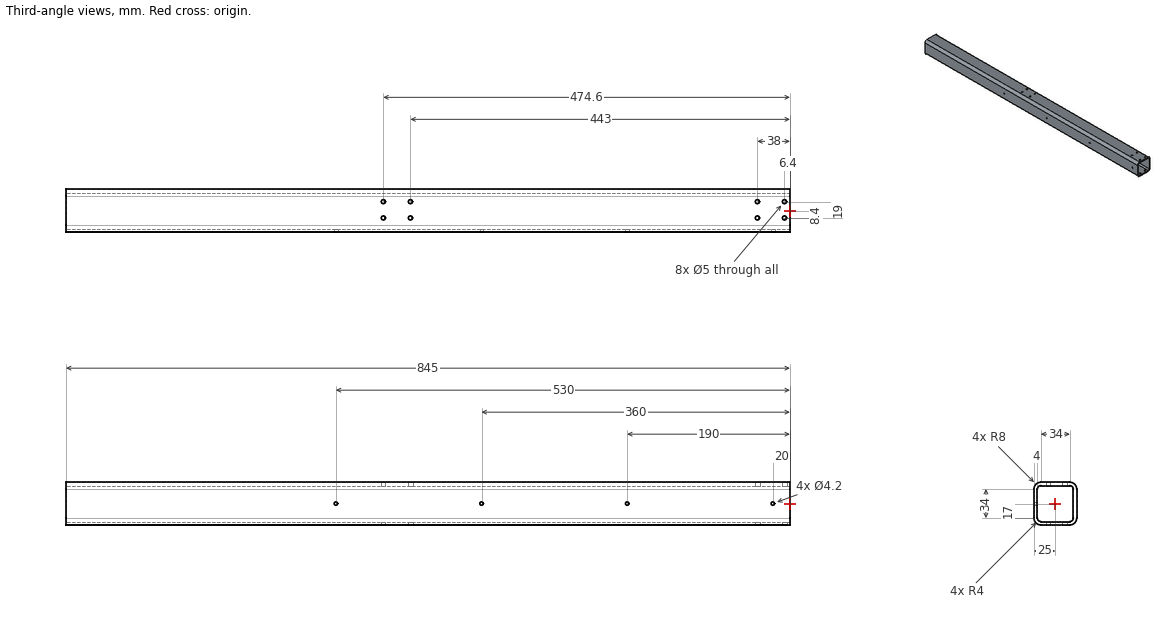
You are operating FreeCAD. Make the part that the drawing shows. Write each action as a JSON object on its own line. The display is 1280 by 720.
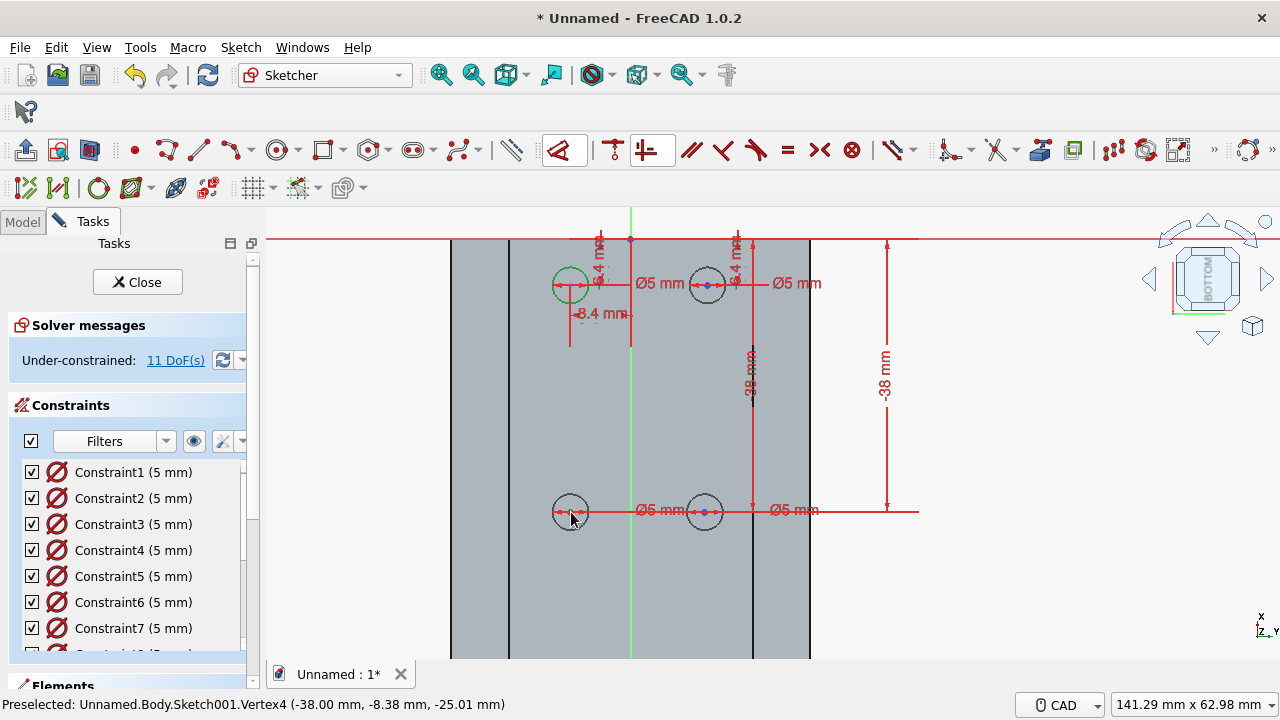
{"action": "left_click", "coordinate": [582, 150]}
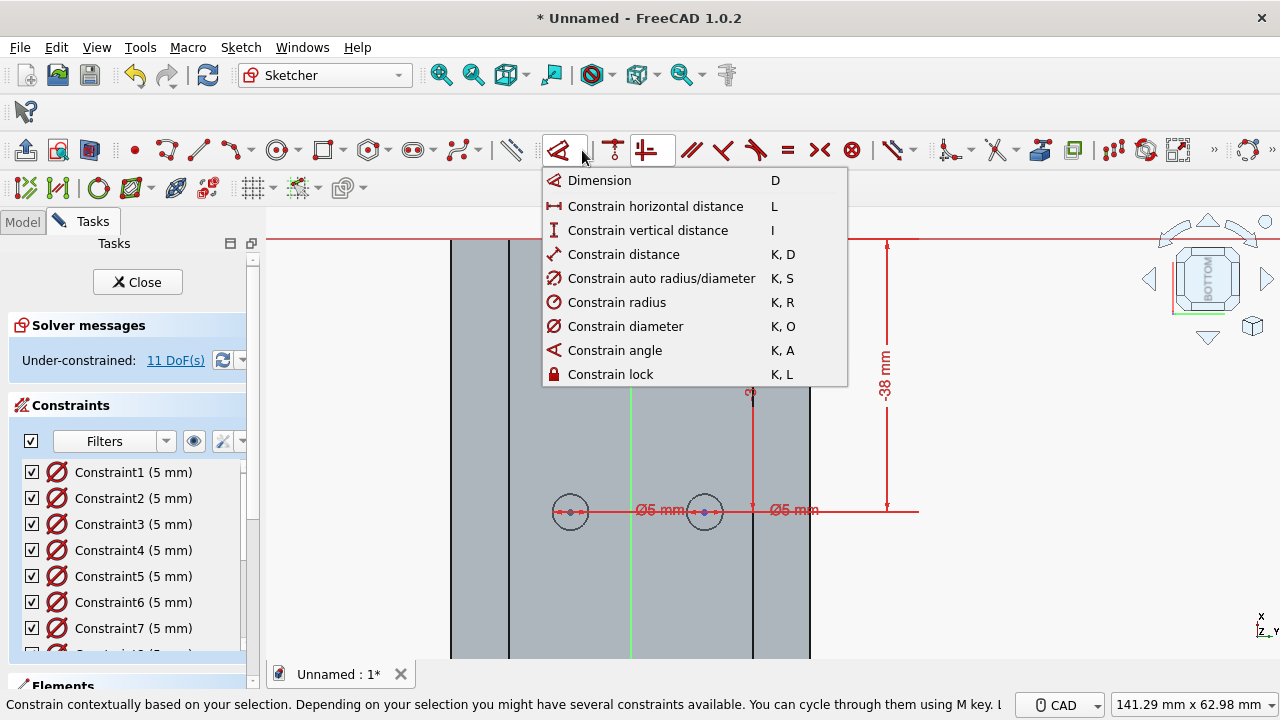
{"action": "left_click", "coordinate": [695, 206]}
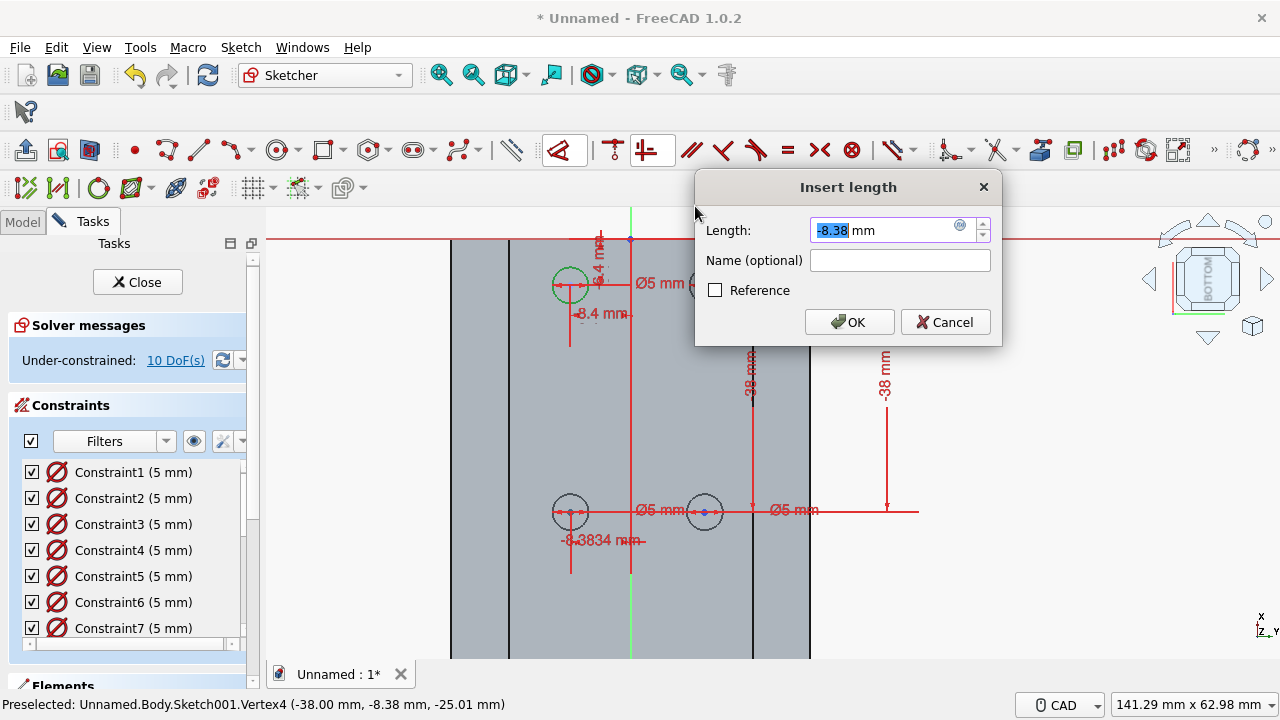
{"action": "type", "text": "-8.4"}
{"action": "key", "text": "Return"}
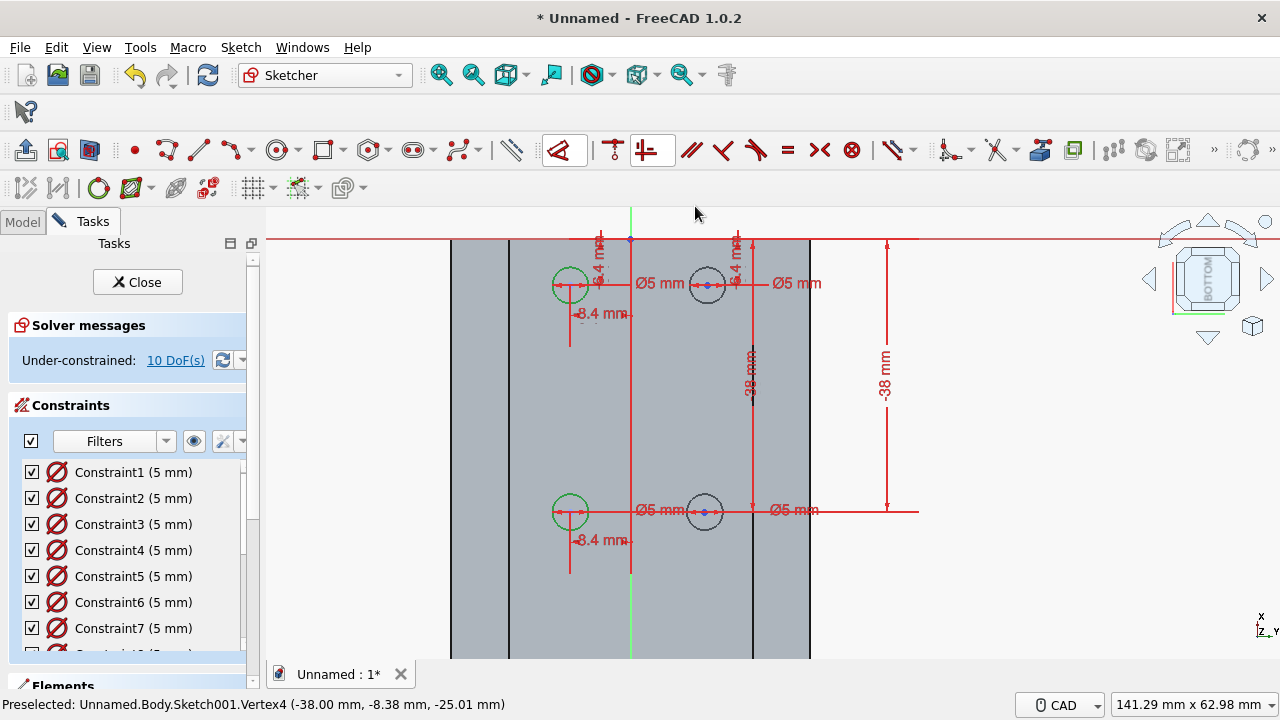
{"action": "scroll", "coordinate": [710, 311], "scroll_direction": "down", "scroll_amount": 13}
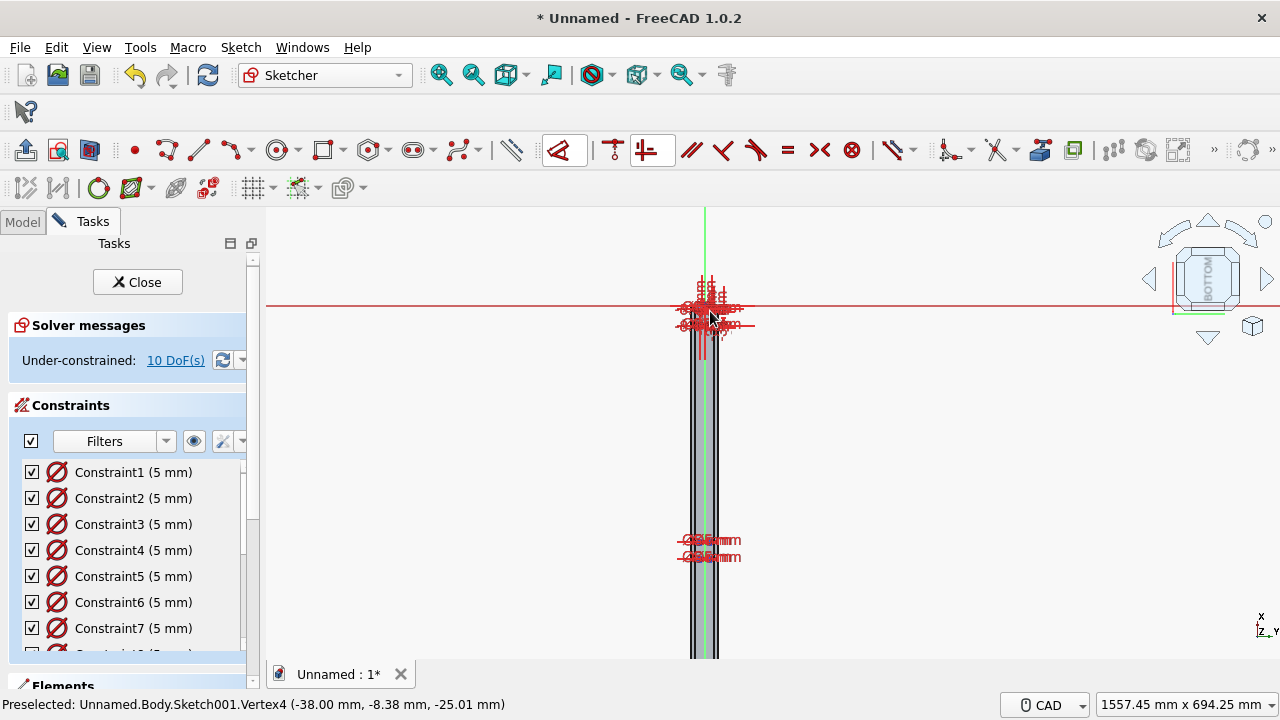
{"action": "left_click", "coordinate": [710, 542]}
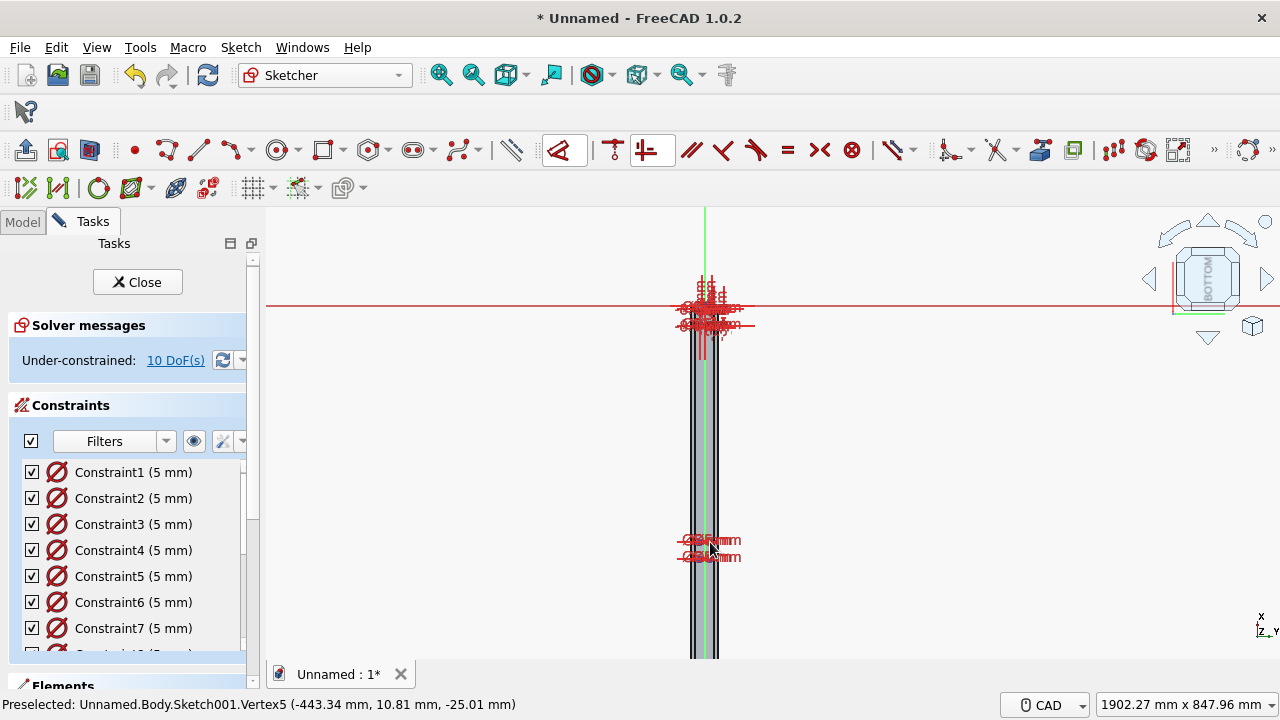
{"action": "left_click", "coordinate": [582, 150]}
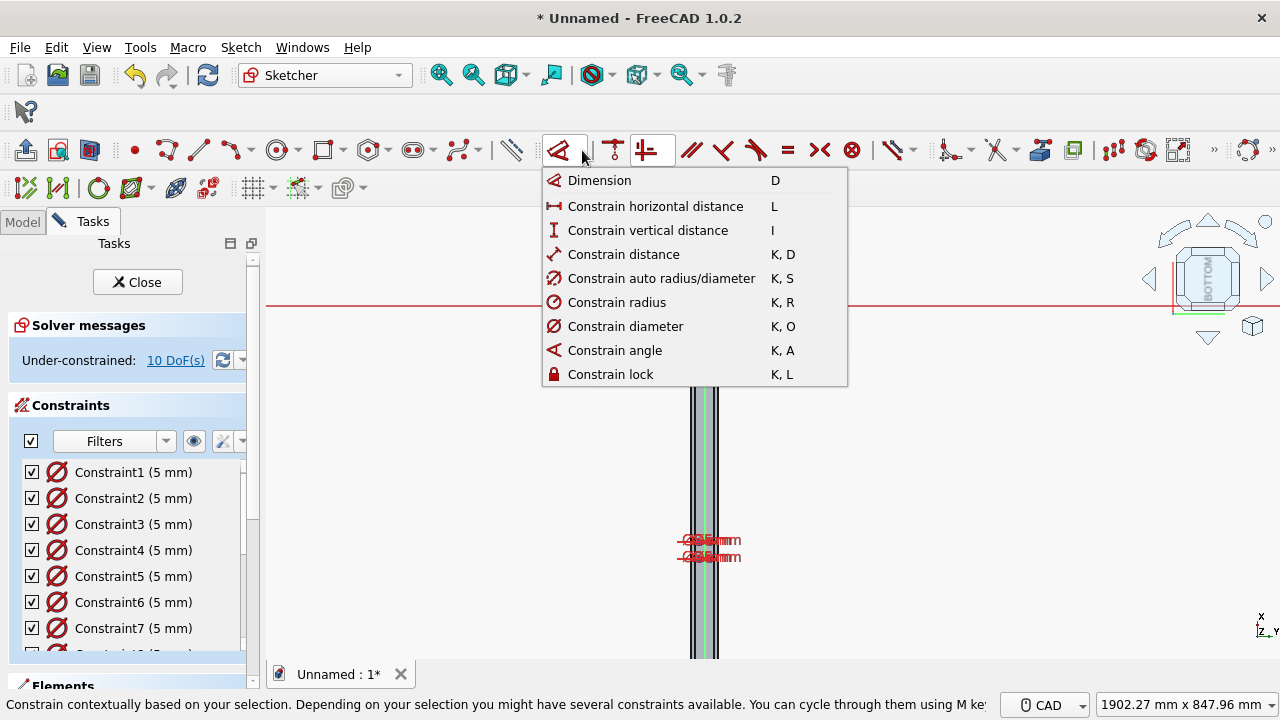
{"action": "left_click", "coordinate": [695, 230]}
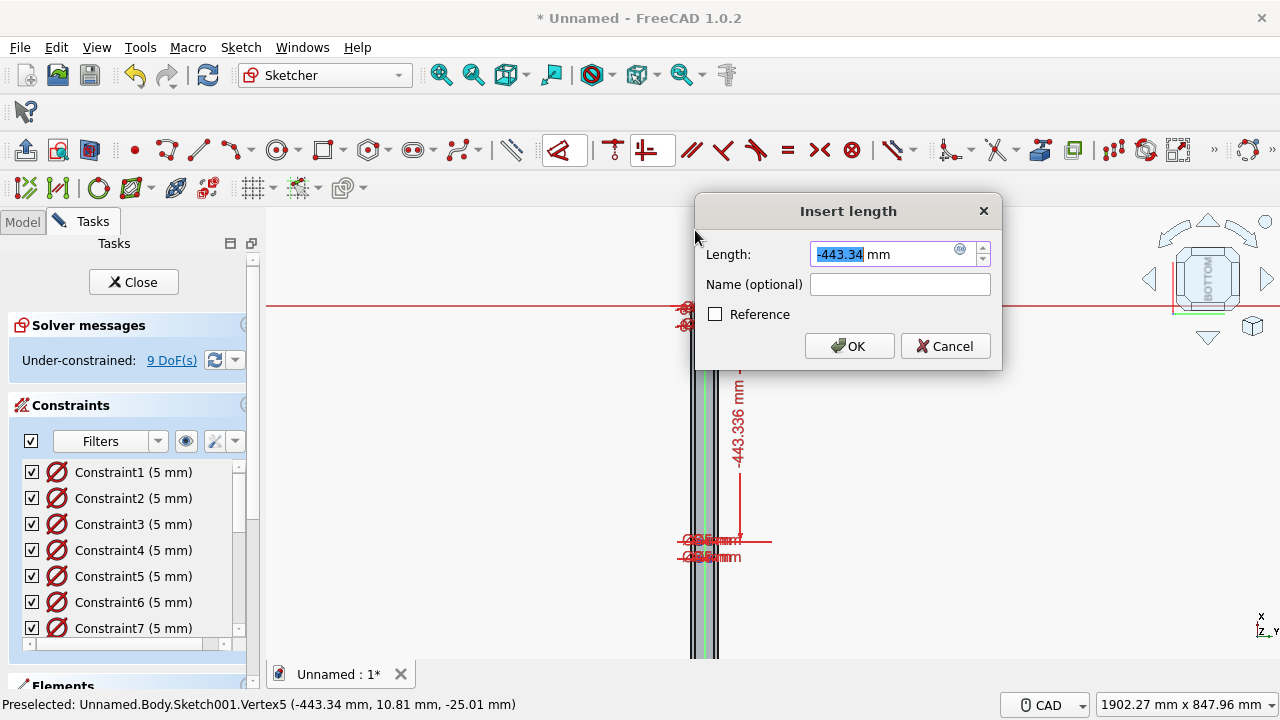
{"action": "type", "text": "-443"}
{"action": "key", "text": "Return"}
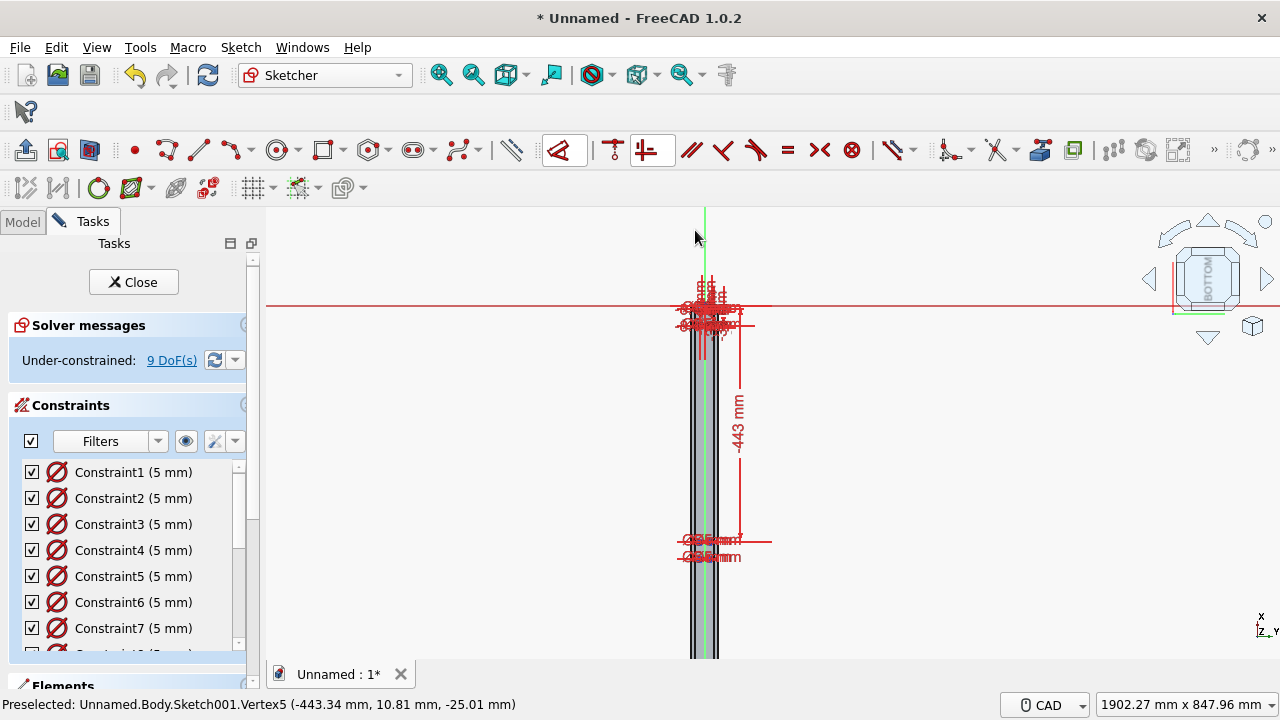
{"action": "scroll", "coordinate": [700, 542], "scroll_direction": "up", "scroll_amount": 11}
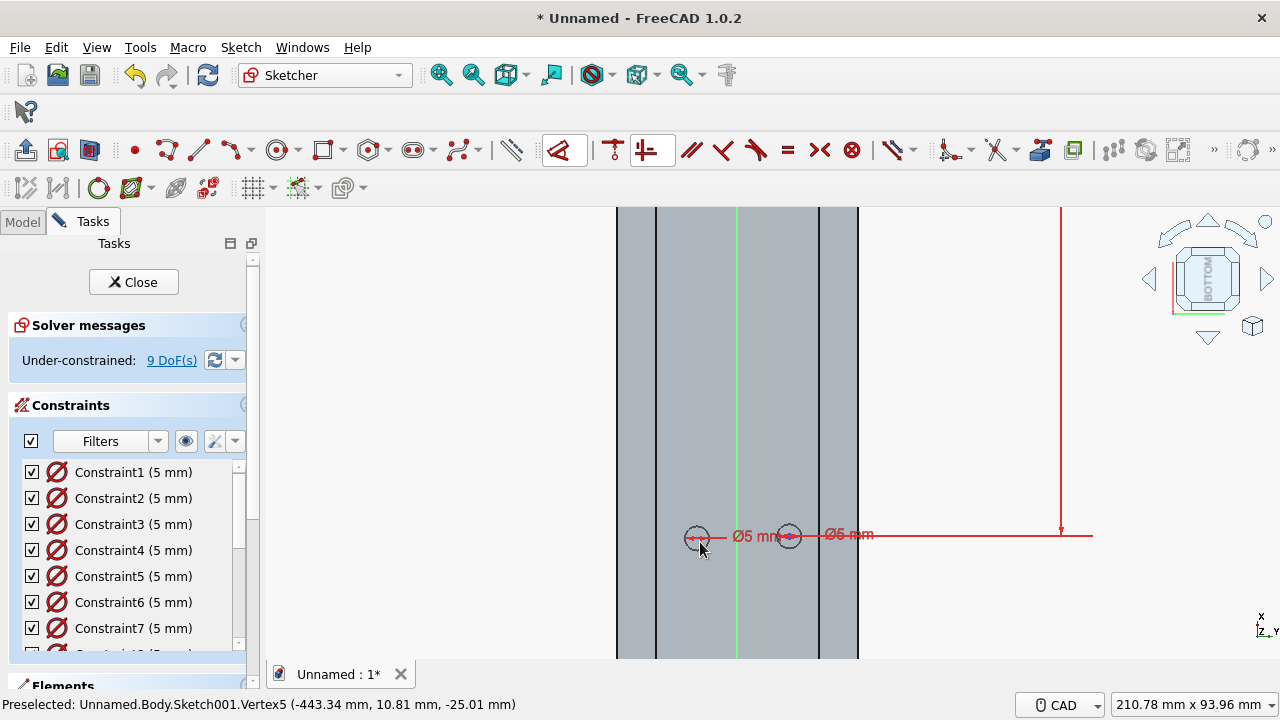
{"action": "left_click", "coordinate": [697, 538]}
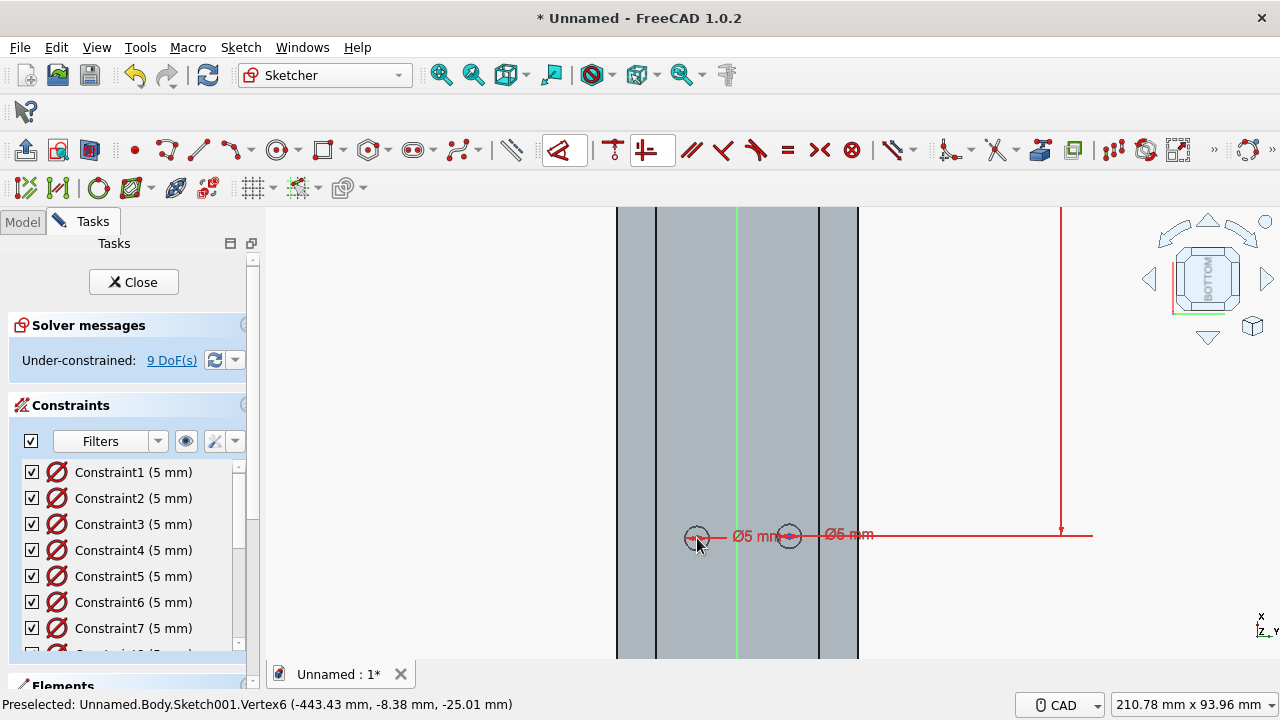
{"action": "left_click", "coordinate": [582, 150]}